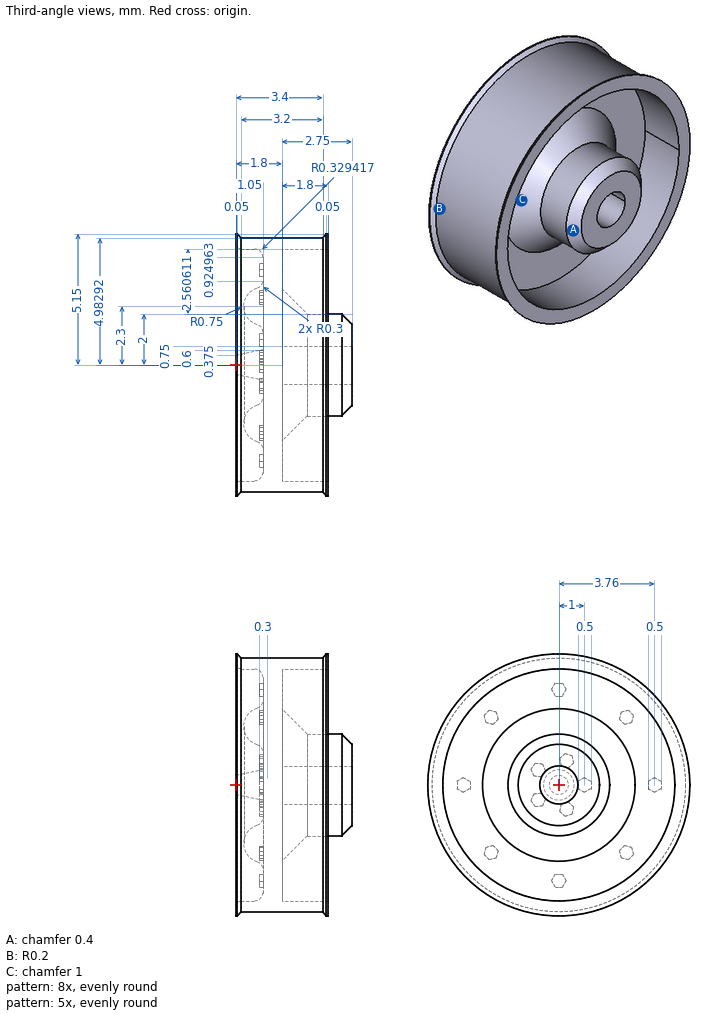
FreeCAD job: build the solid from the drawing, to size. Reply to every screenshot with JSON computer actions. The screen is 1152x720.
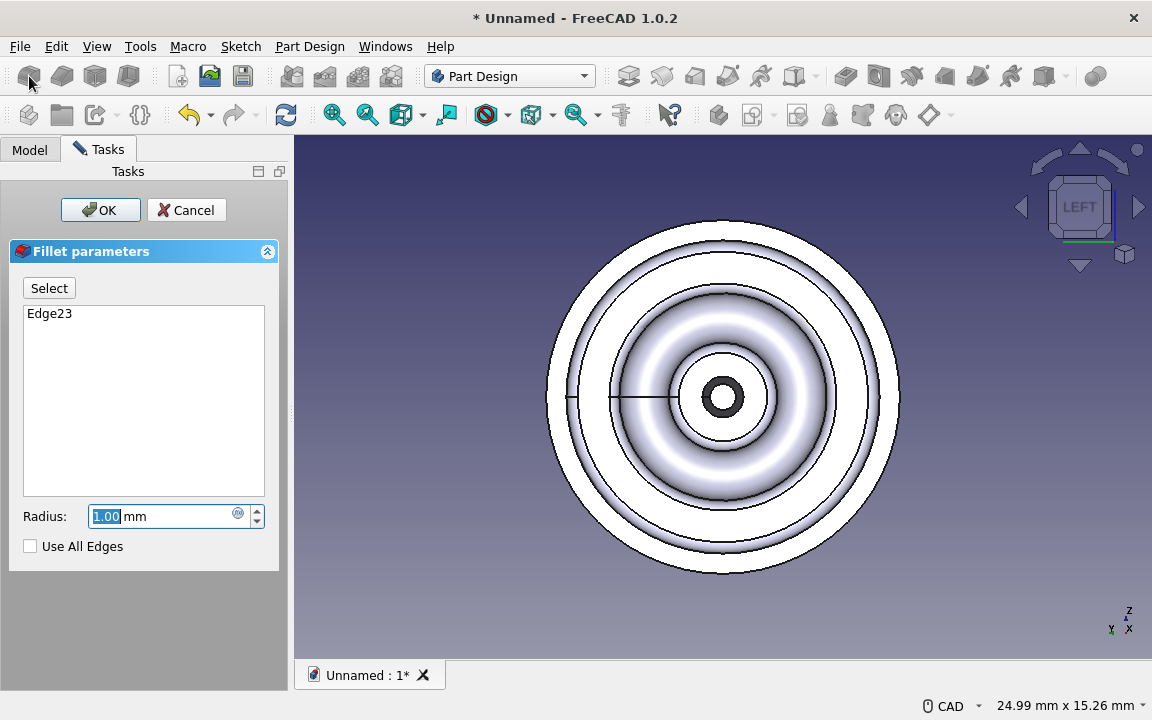
{"action": "type", "text": "0.2"}
{"action": "key", "text": "Tab"}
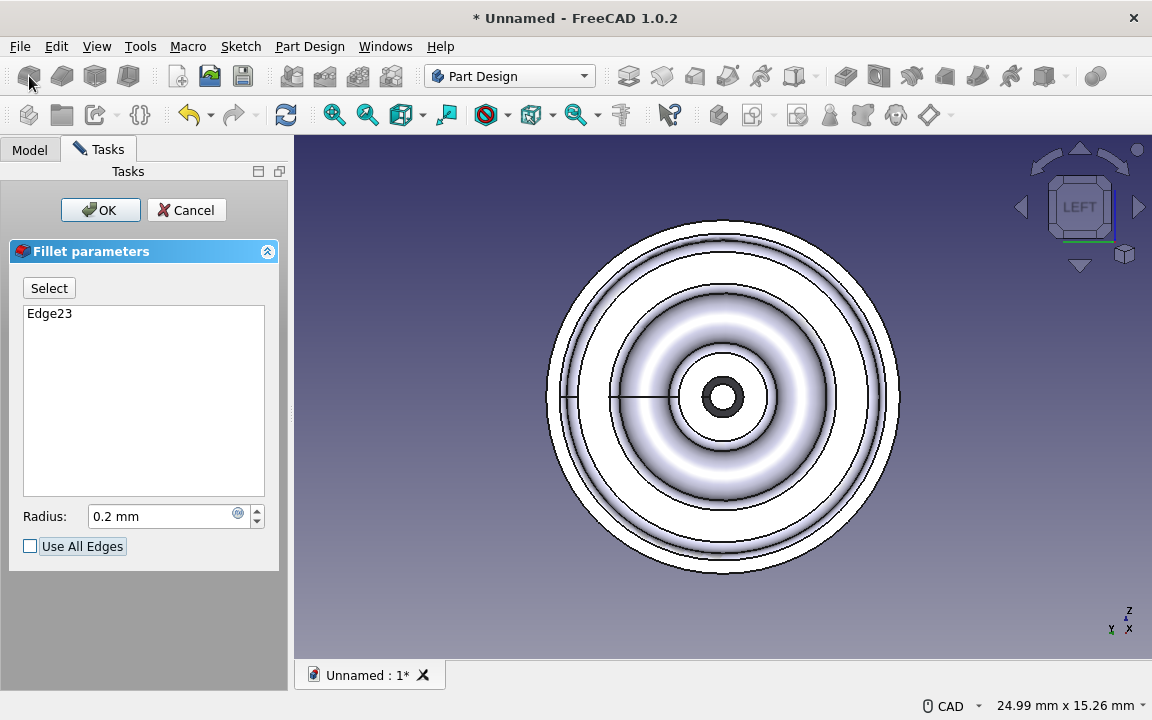
{"action": "left_click", "coordinate": [101, 210]}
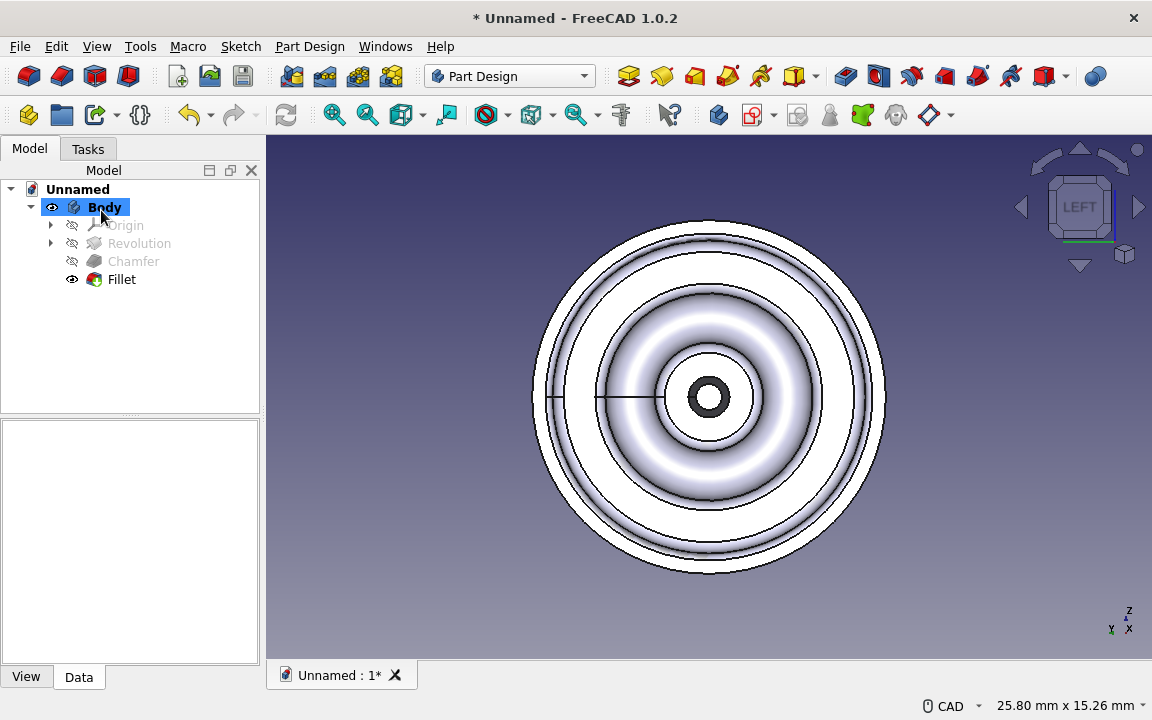
{"action": "key", "text": "0"}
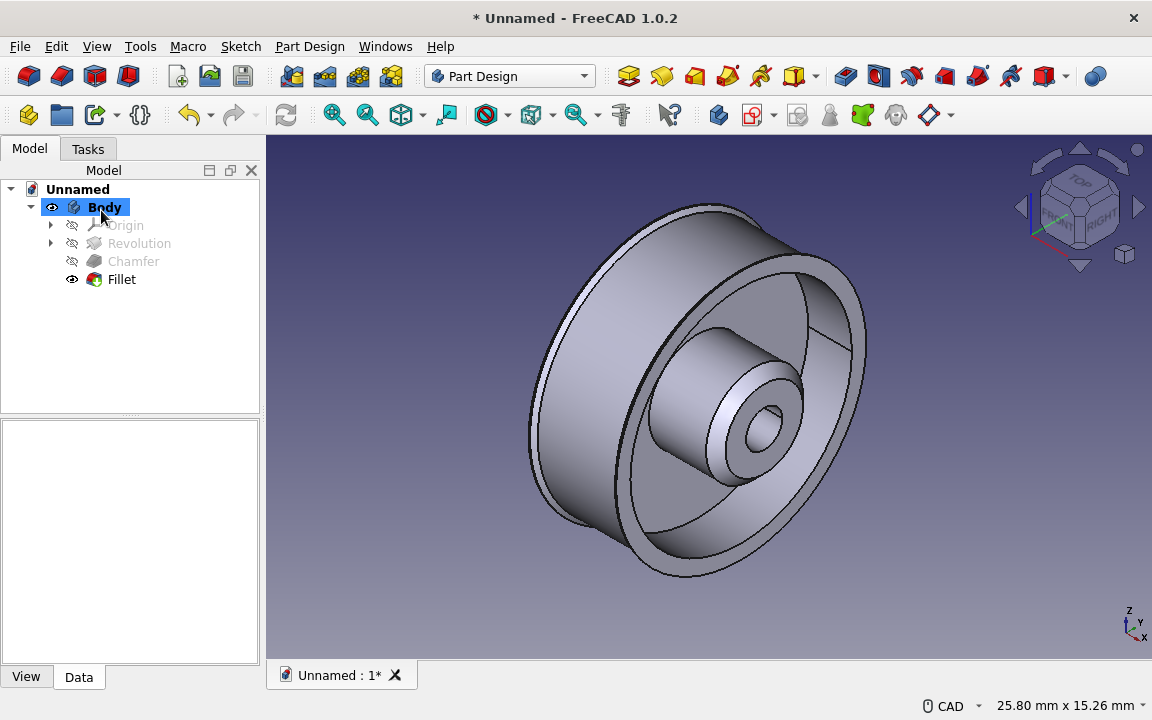
{"action": "key", "text": "2"}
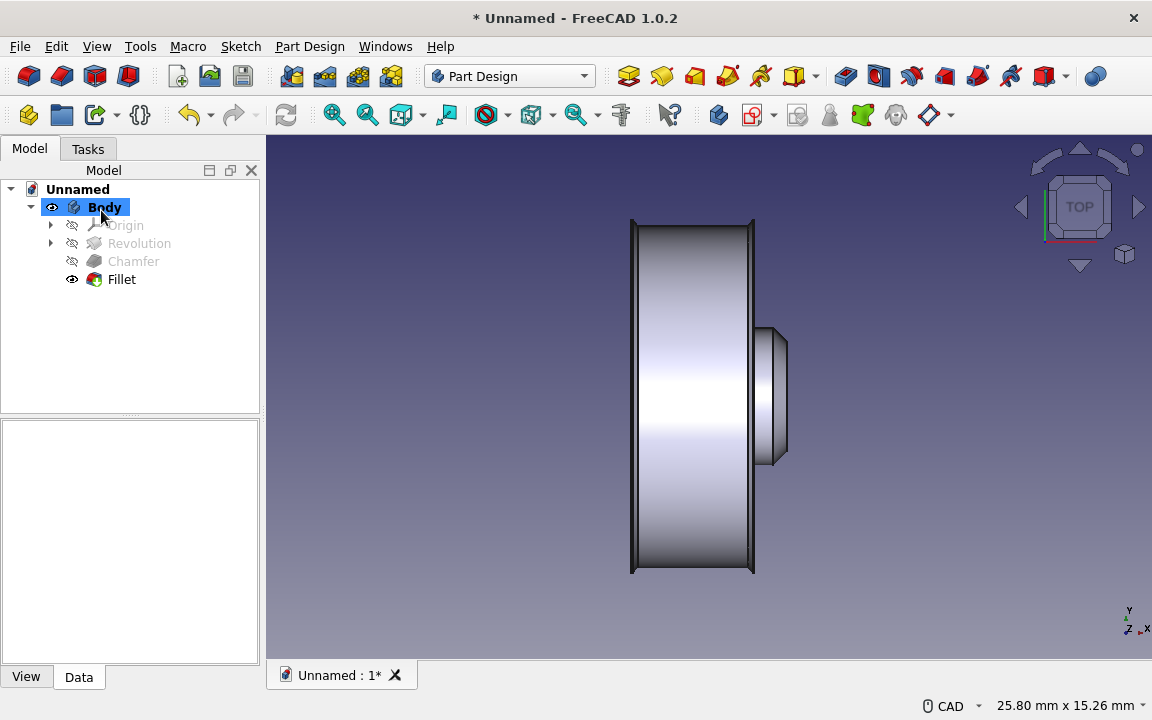
{"action": "key", "text": "1"}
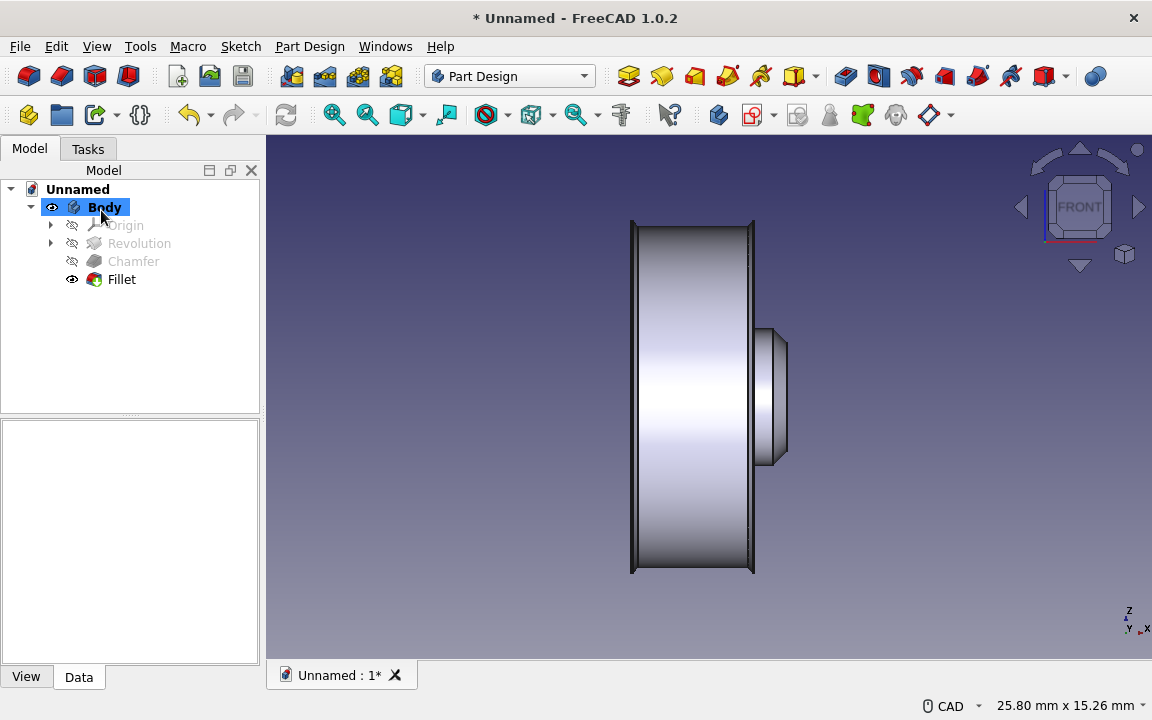
{"action": "key", "text": "3"}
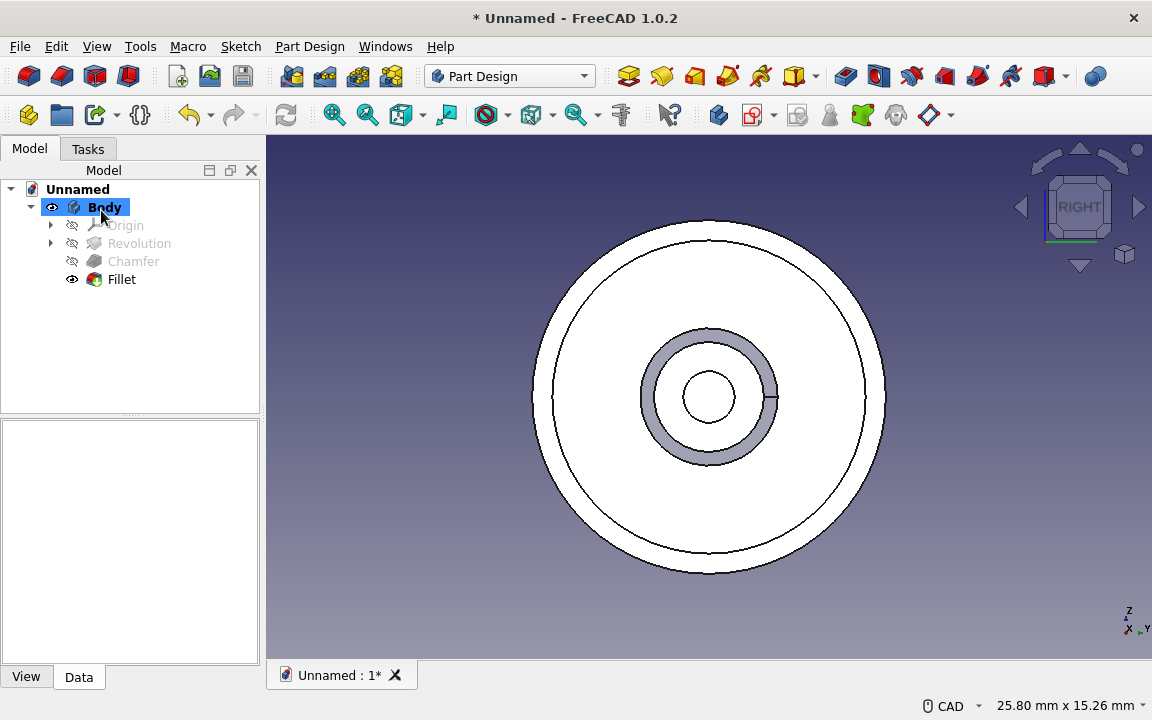
{"action": "key", "text": "5"}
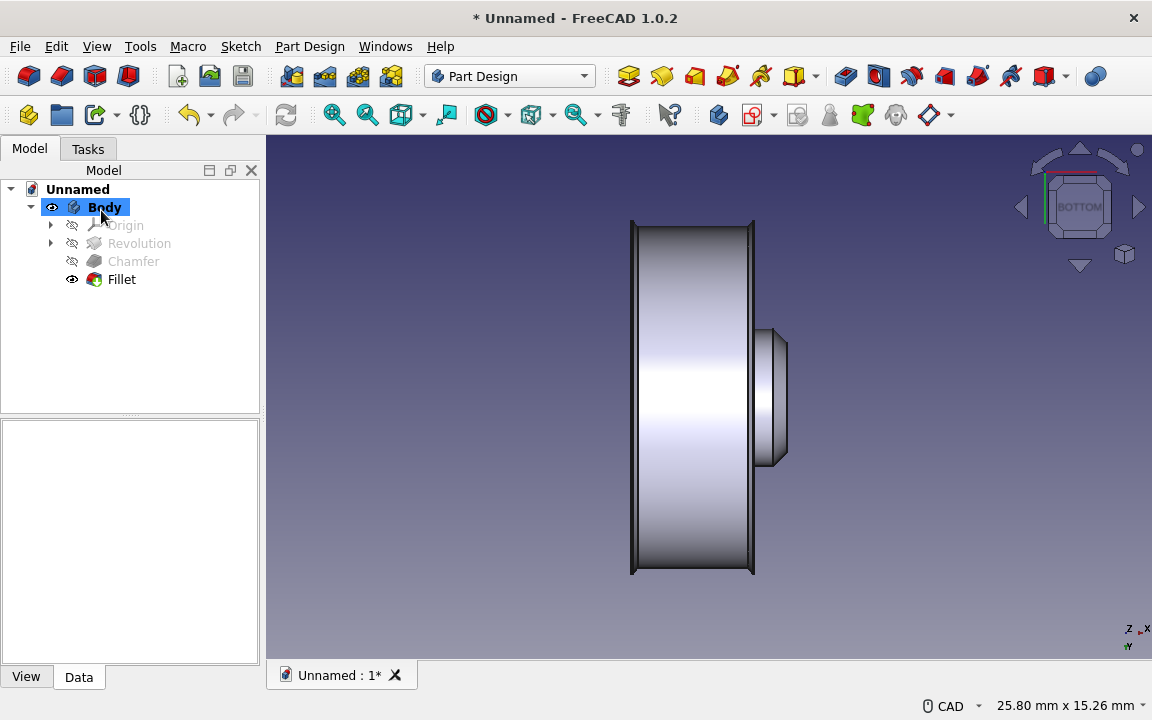
{"action": "key", "text": "4"}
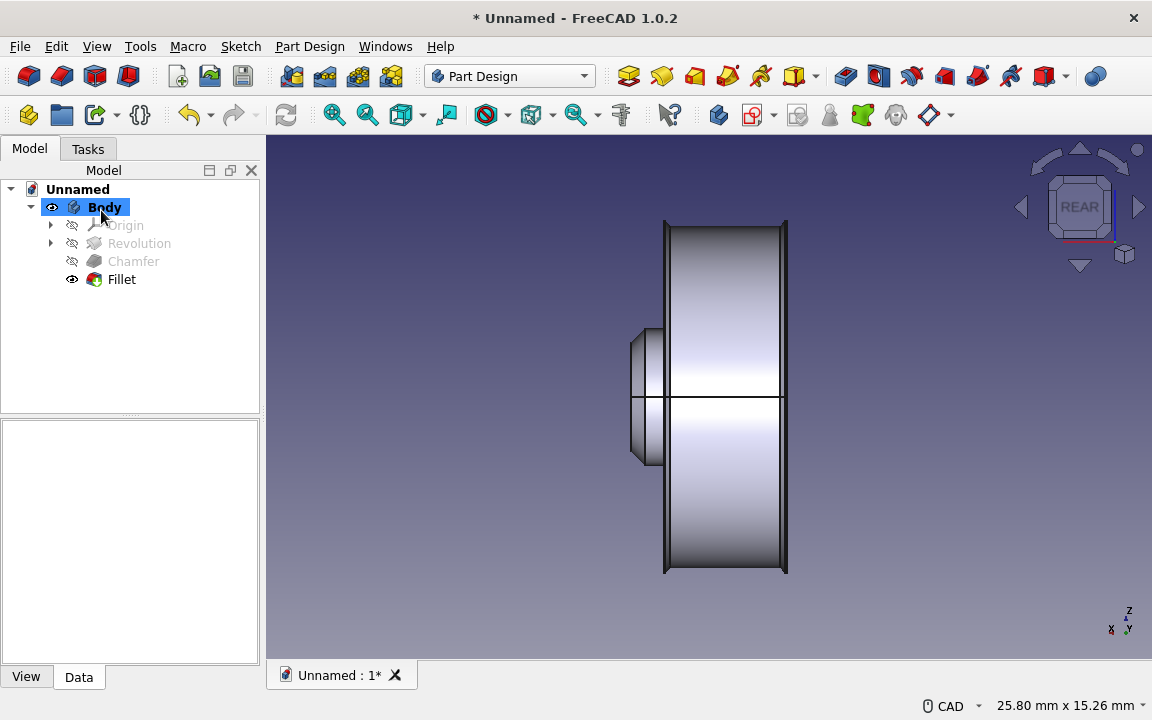
{"action": "key", "text": "6"}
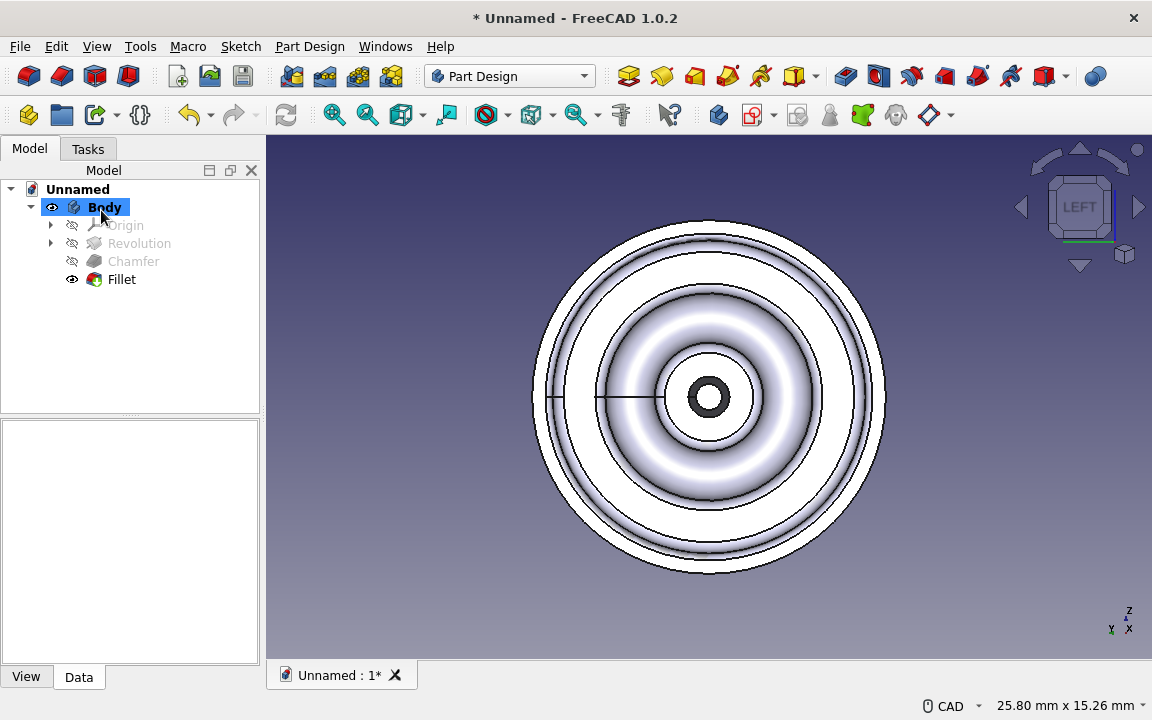
{"action": "key", "text": "v 3"}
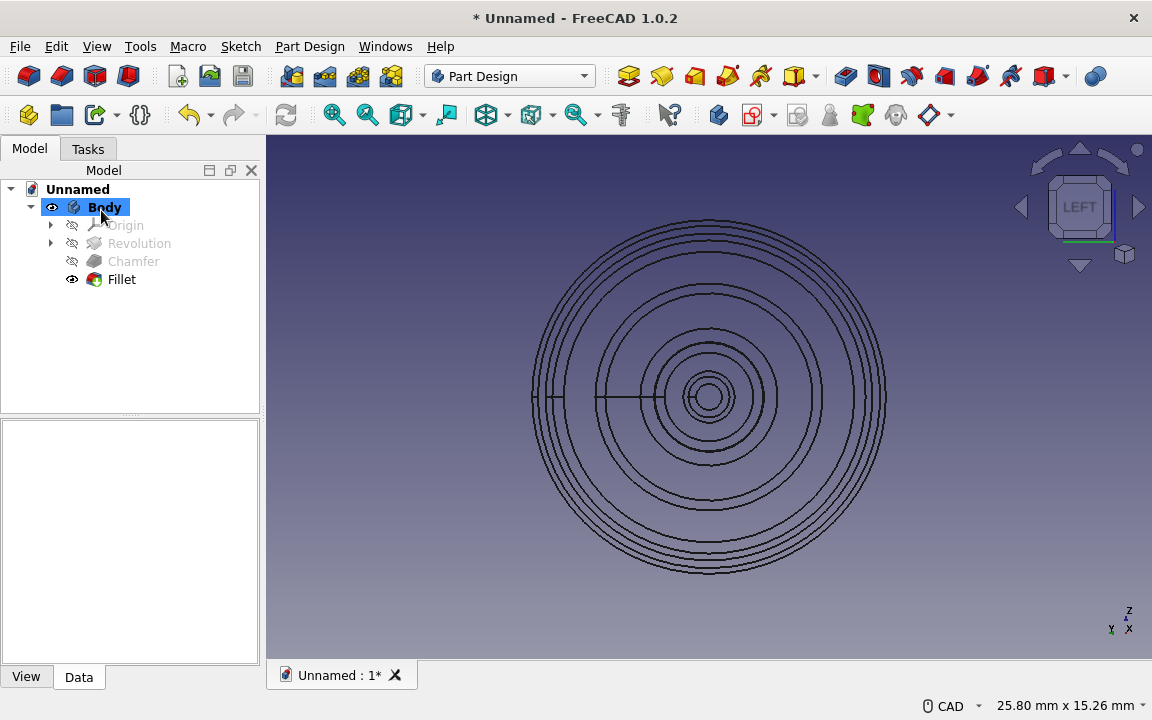
{"action": "key", "text": "0"}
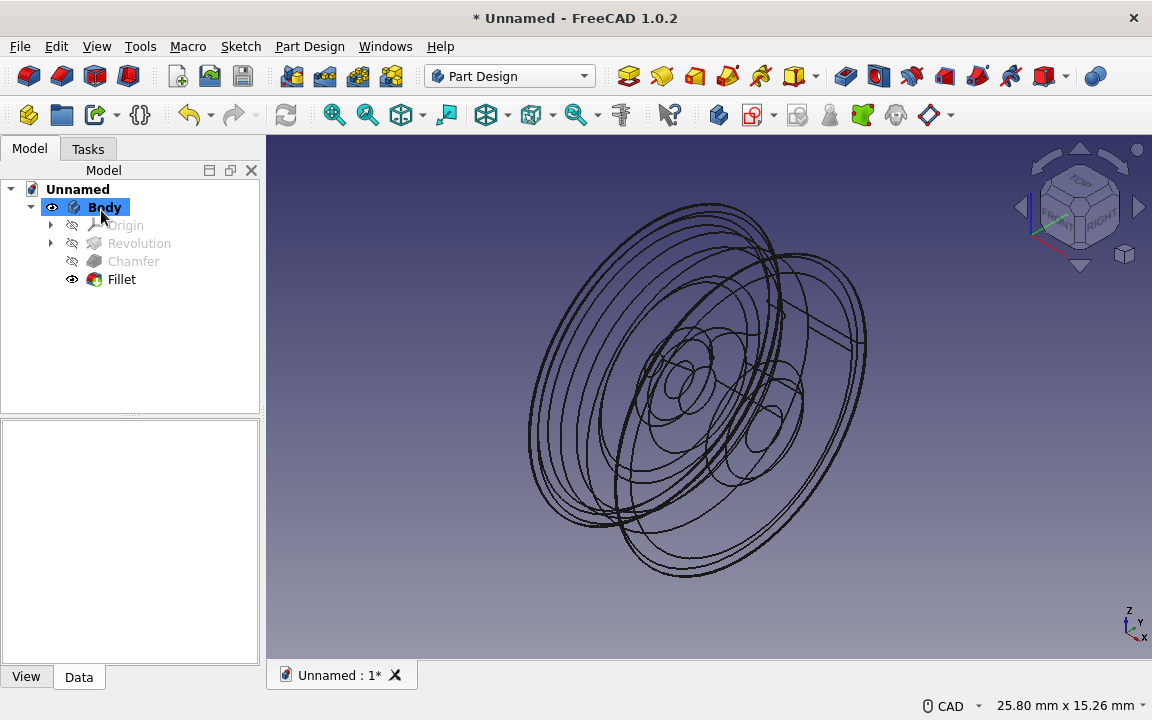
{"action": "left_click", "coordinate": [649, 417]}